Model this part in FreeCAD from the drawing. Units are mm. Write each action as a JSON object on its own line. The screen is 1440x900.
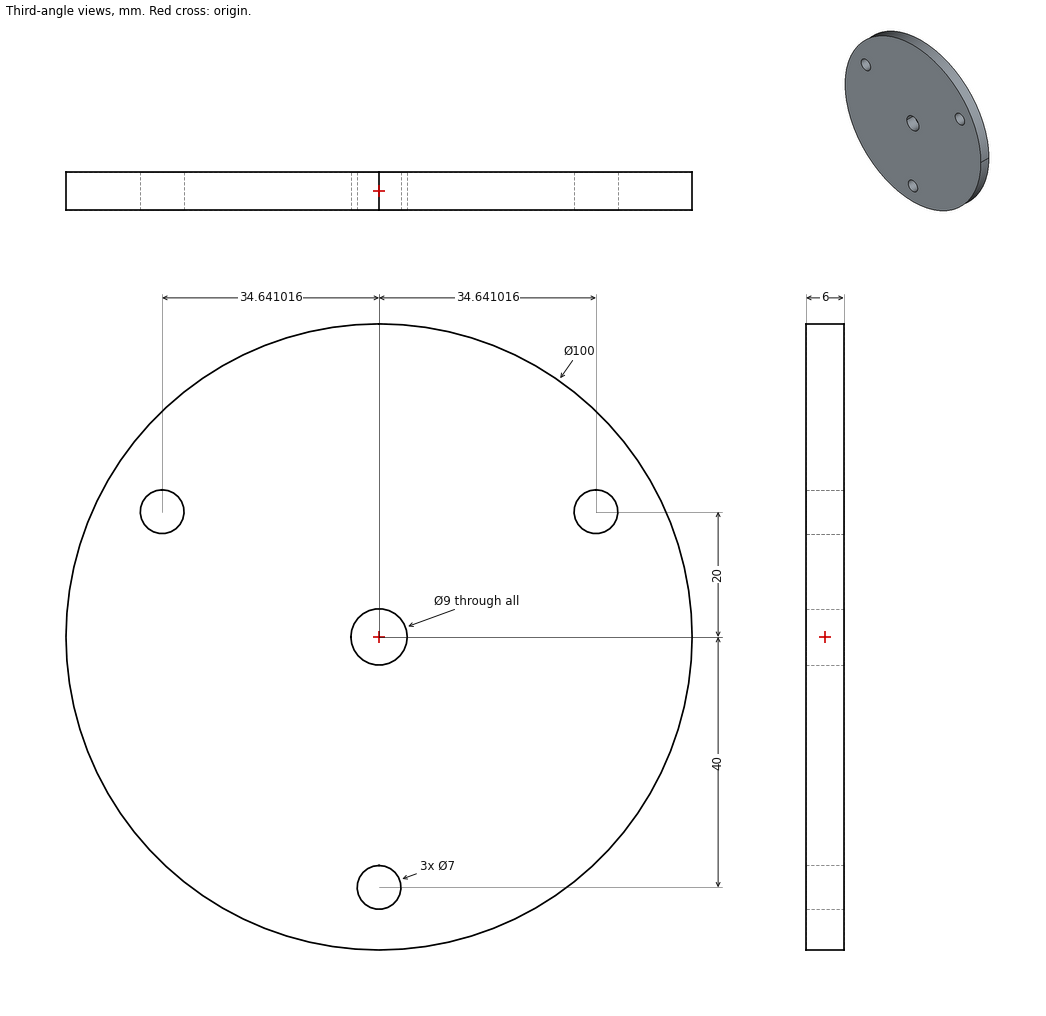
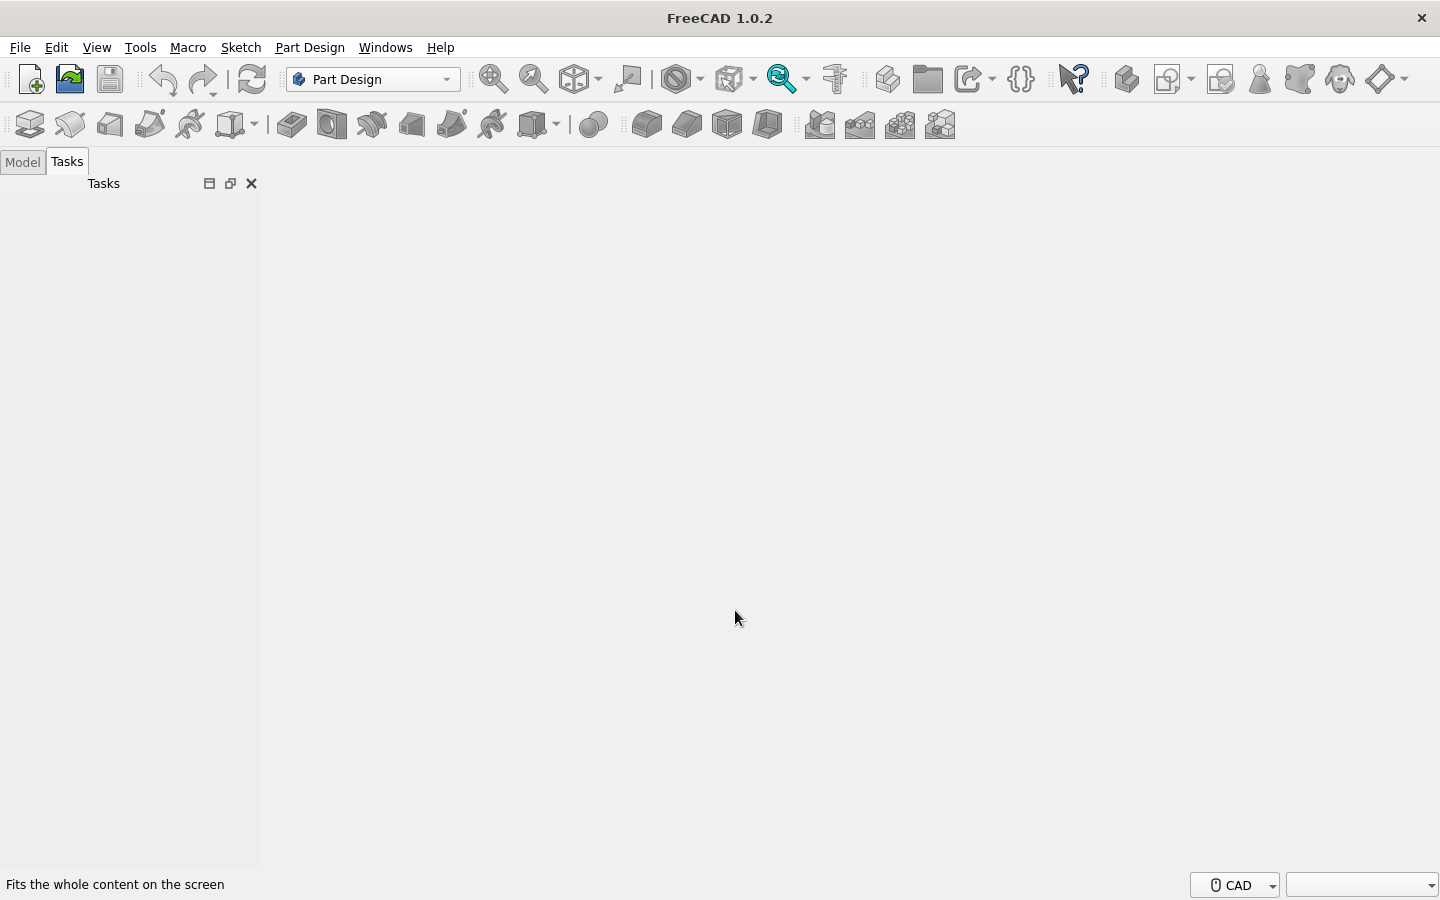
{"action": "left_click", "coordinate": [30, 80]}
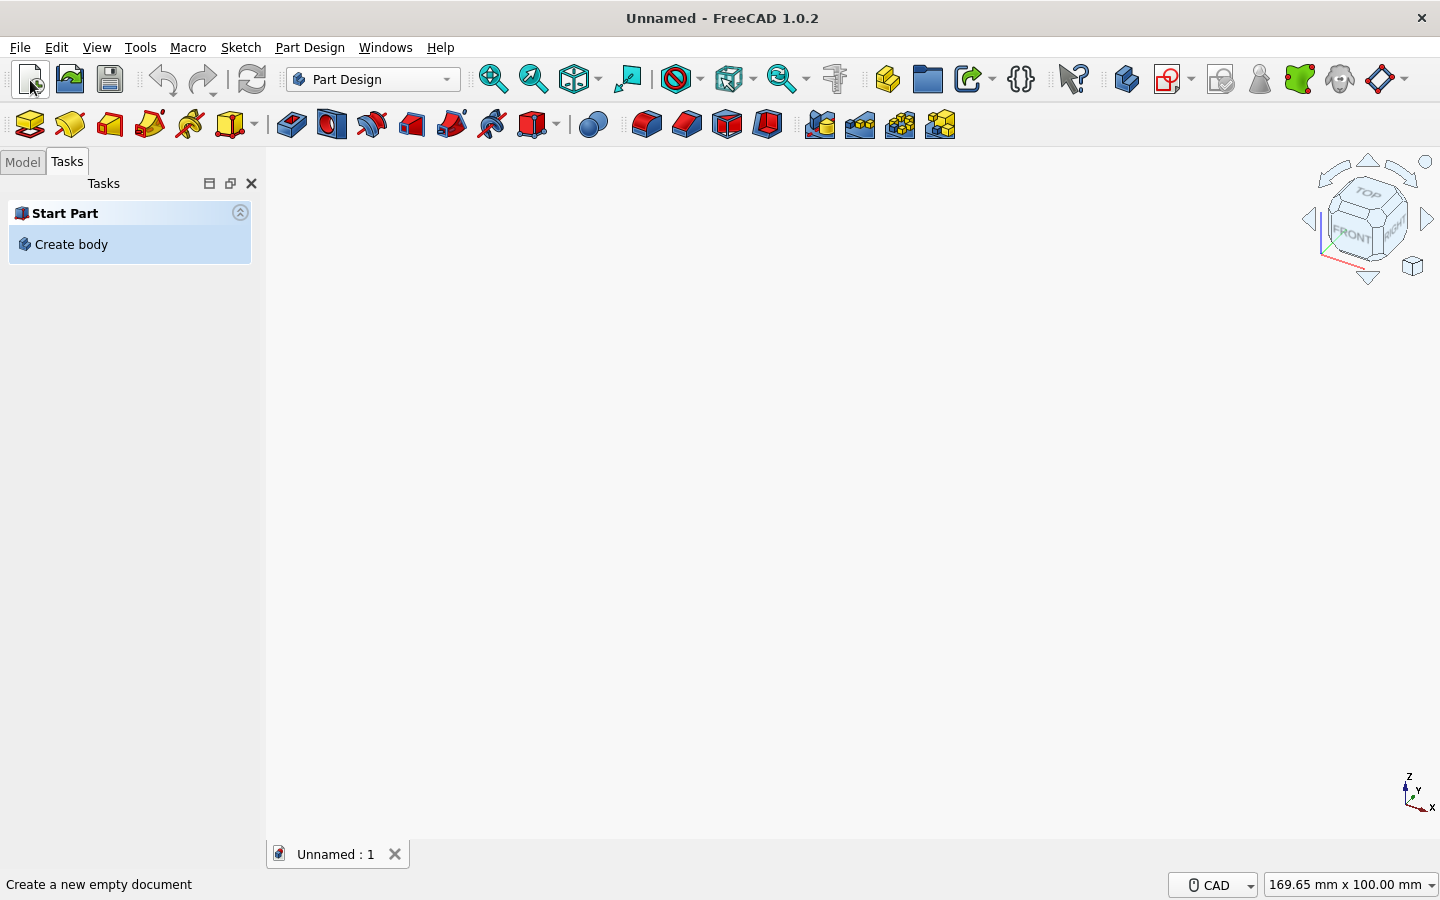
{"action": "left_click", "coordinate": [1168, 80]}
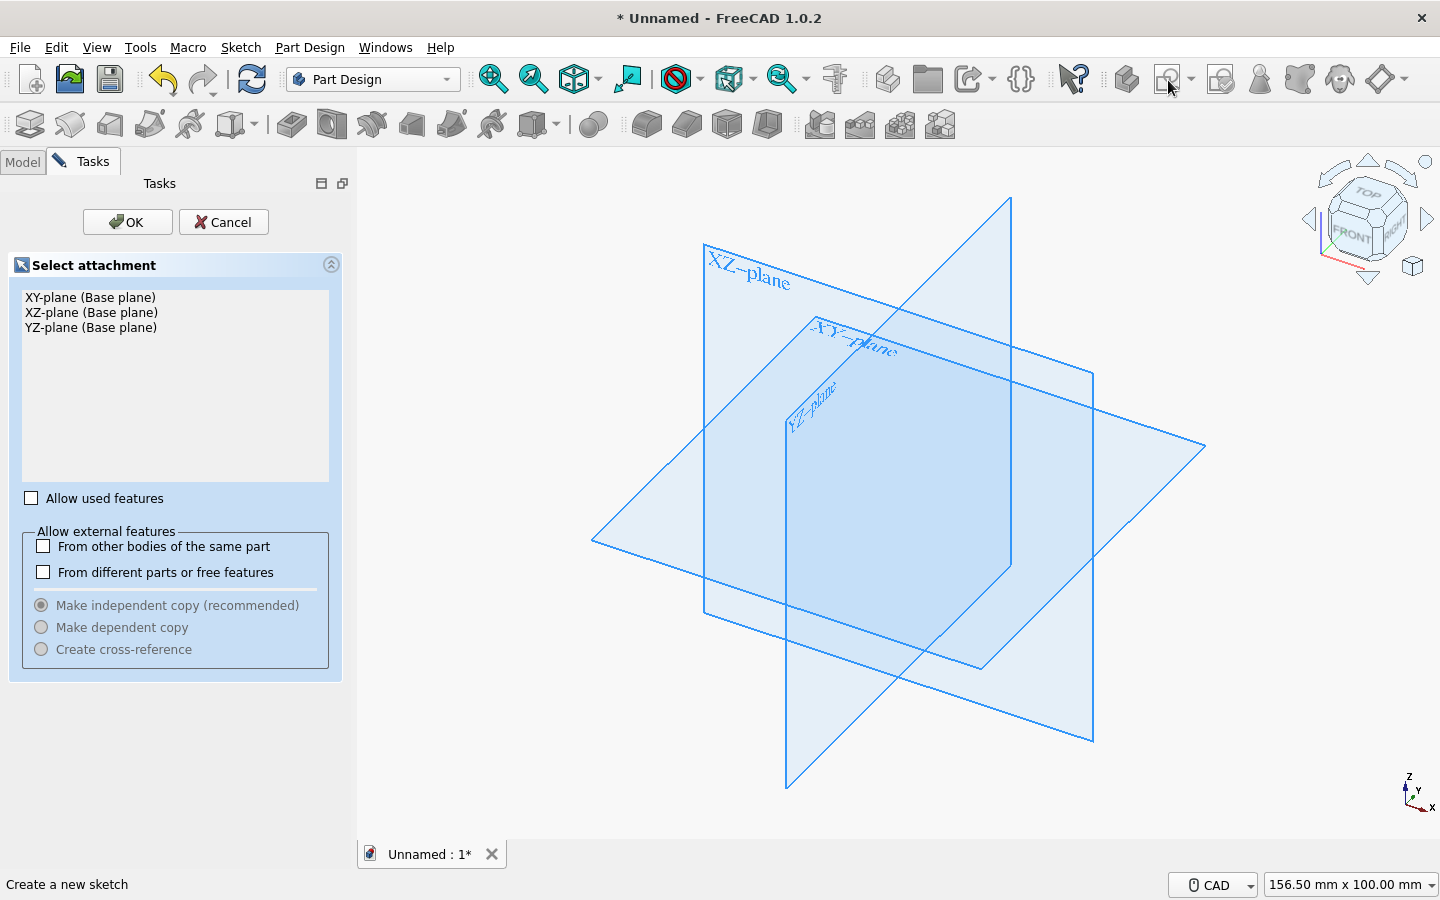
{"action": "left_click", "coordinate": [82, 312]}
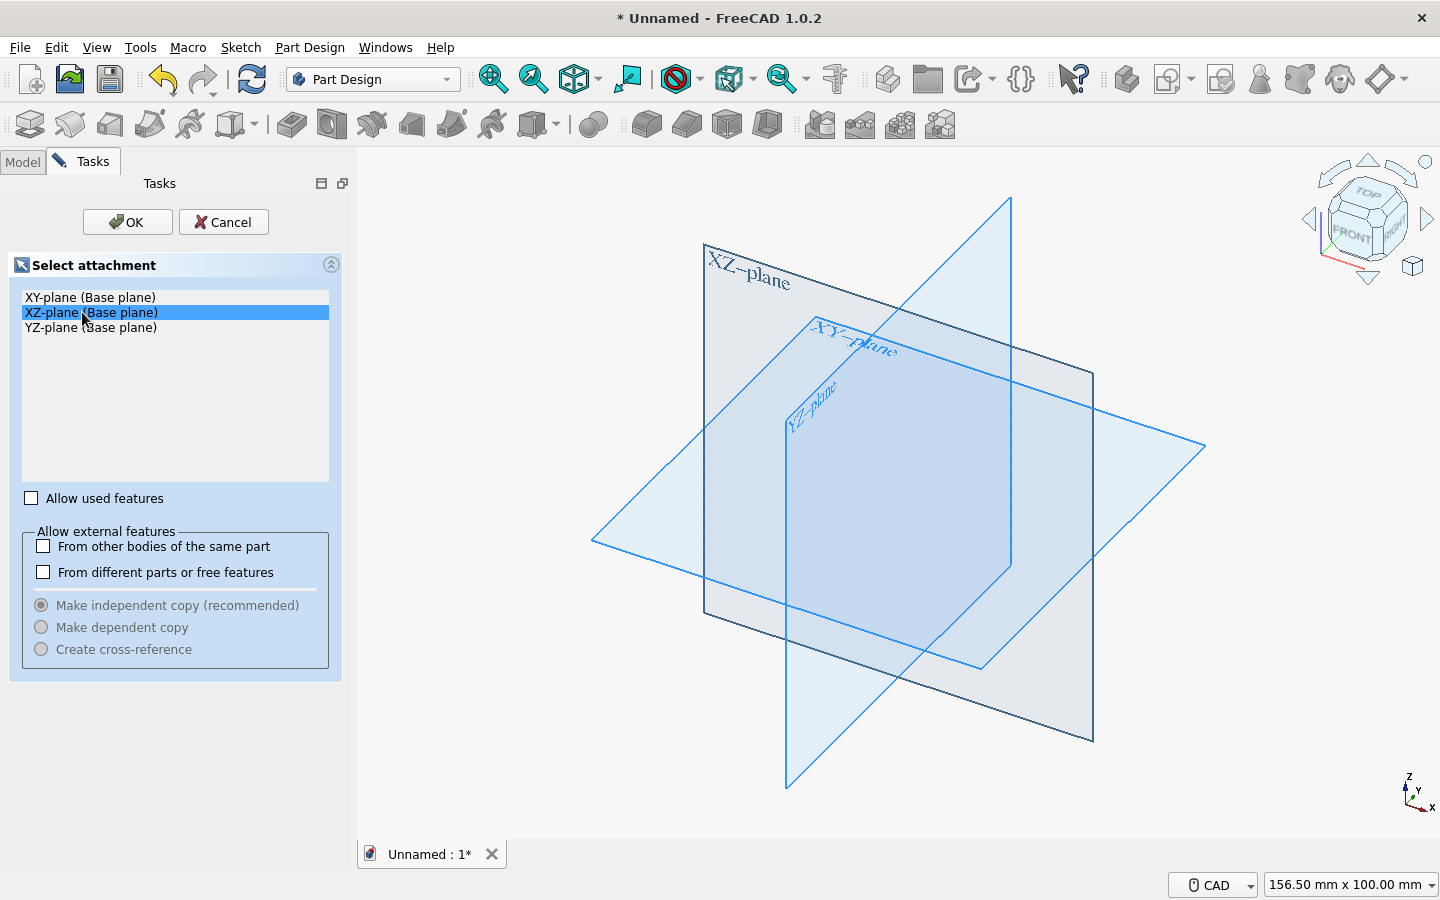
{"action": "left_click", "coordinate": [128, 222]}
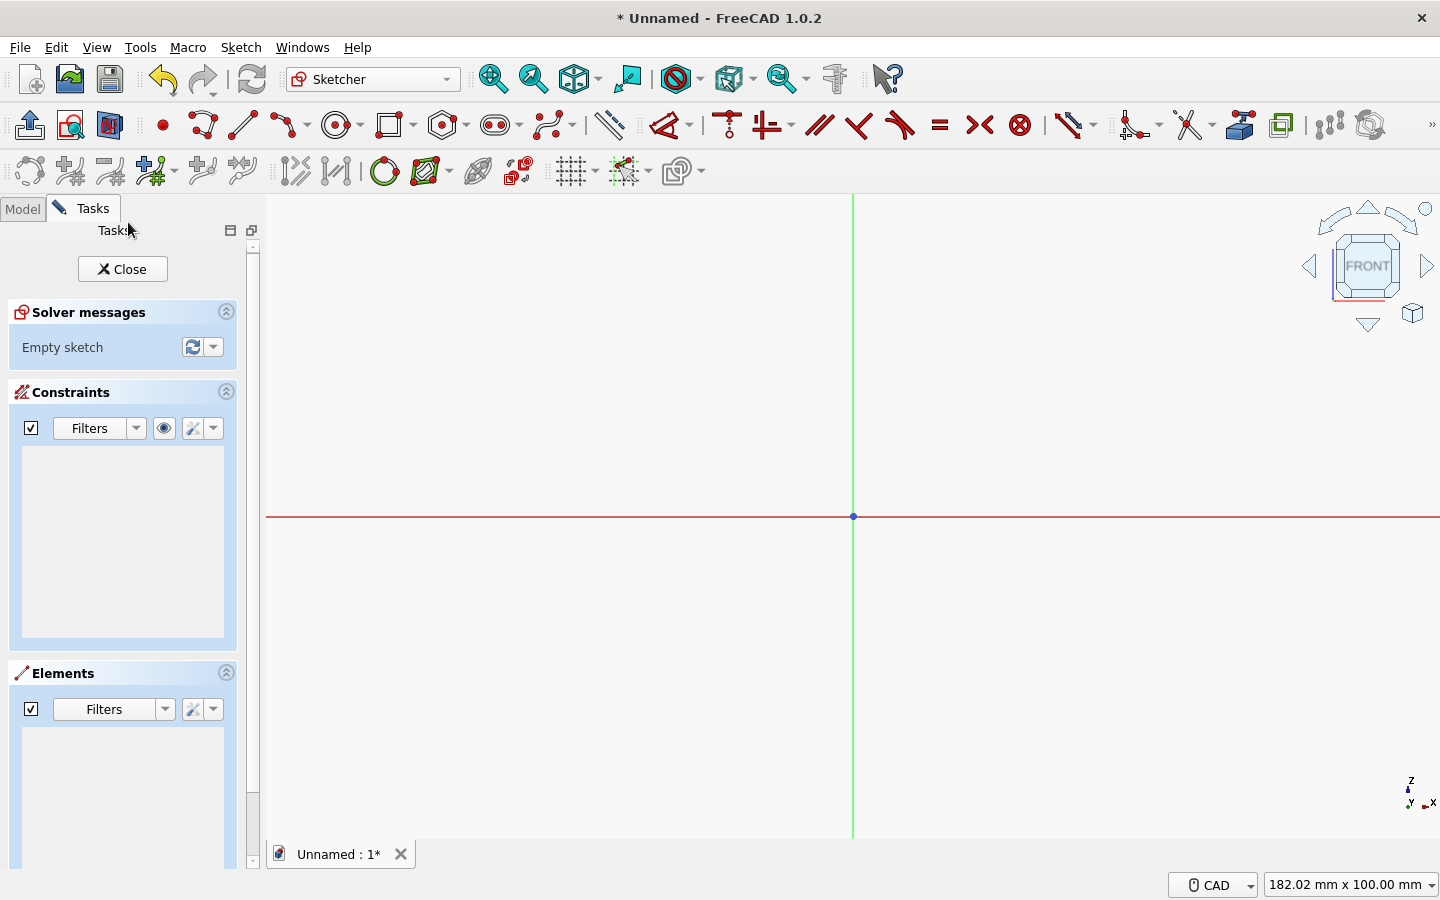
{"action": "scroll", "coordinate": [645, 516], "scroll_direction": "down", "scroll_amount": 2}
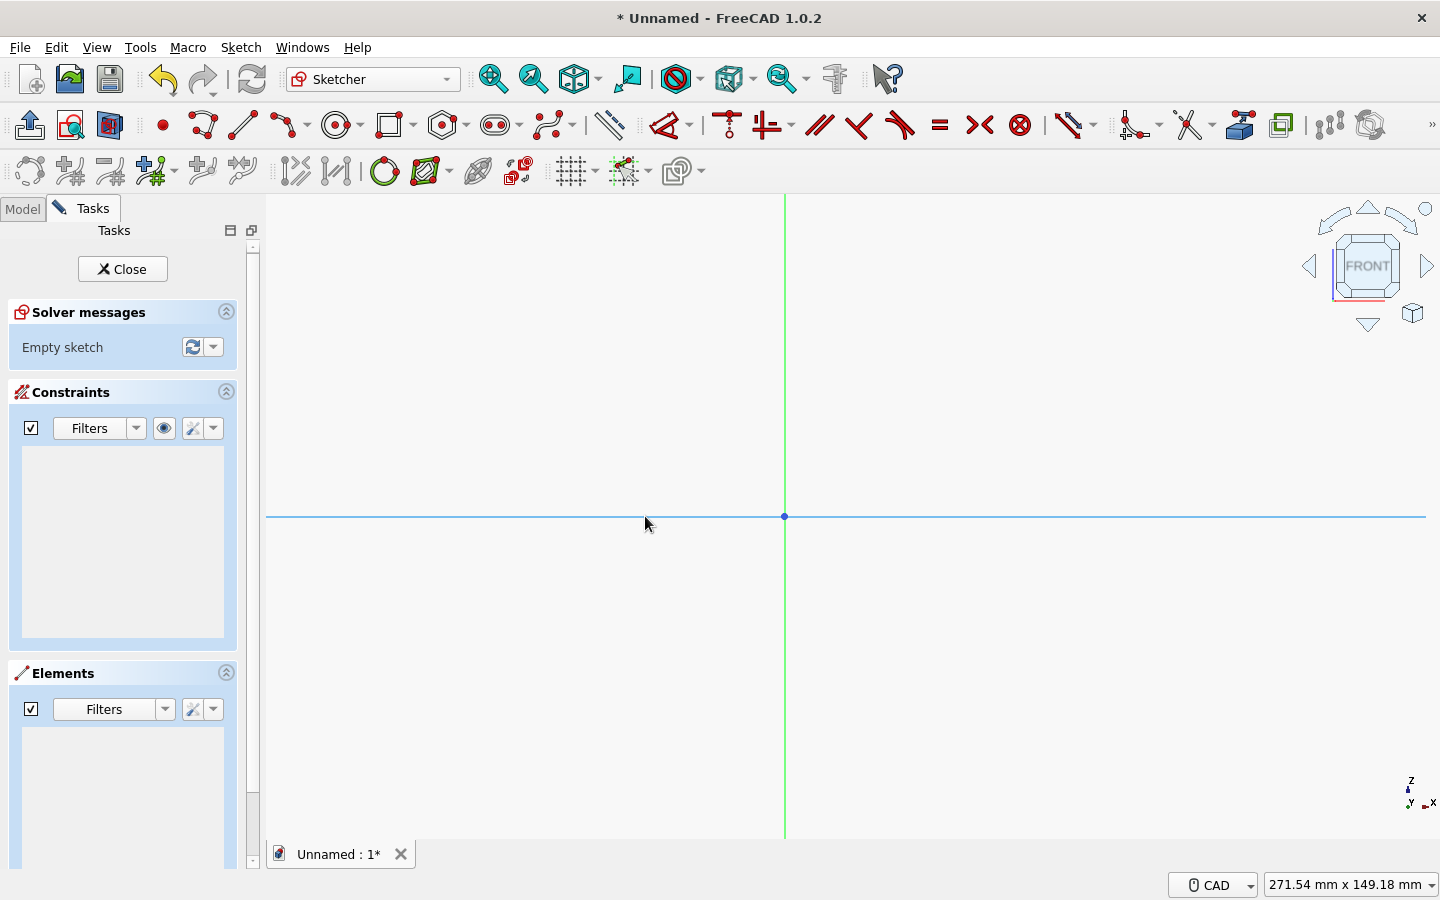
{"action": "left_click", "coordinate": [336, 126]}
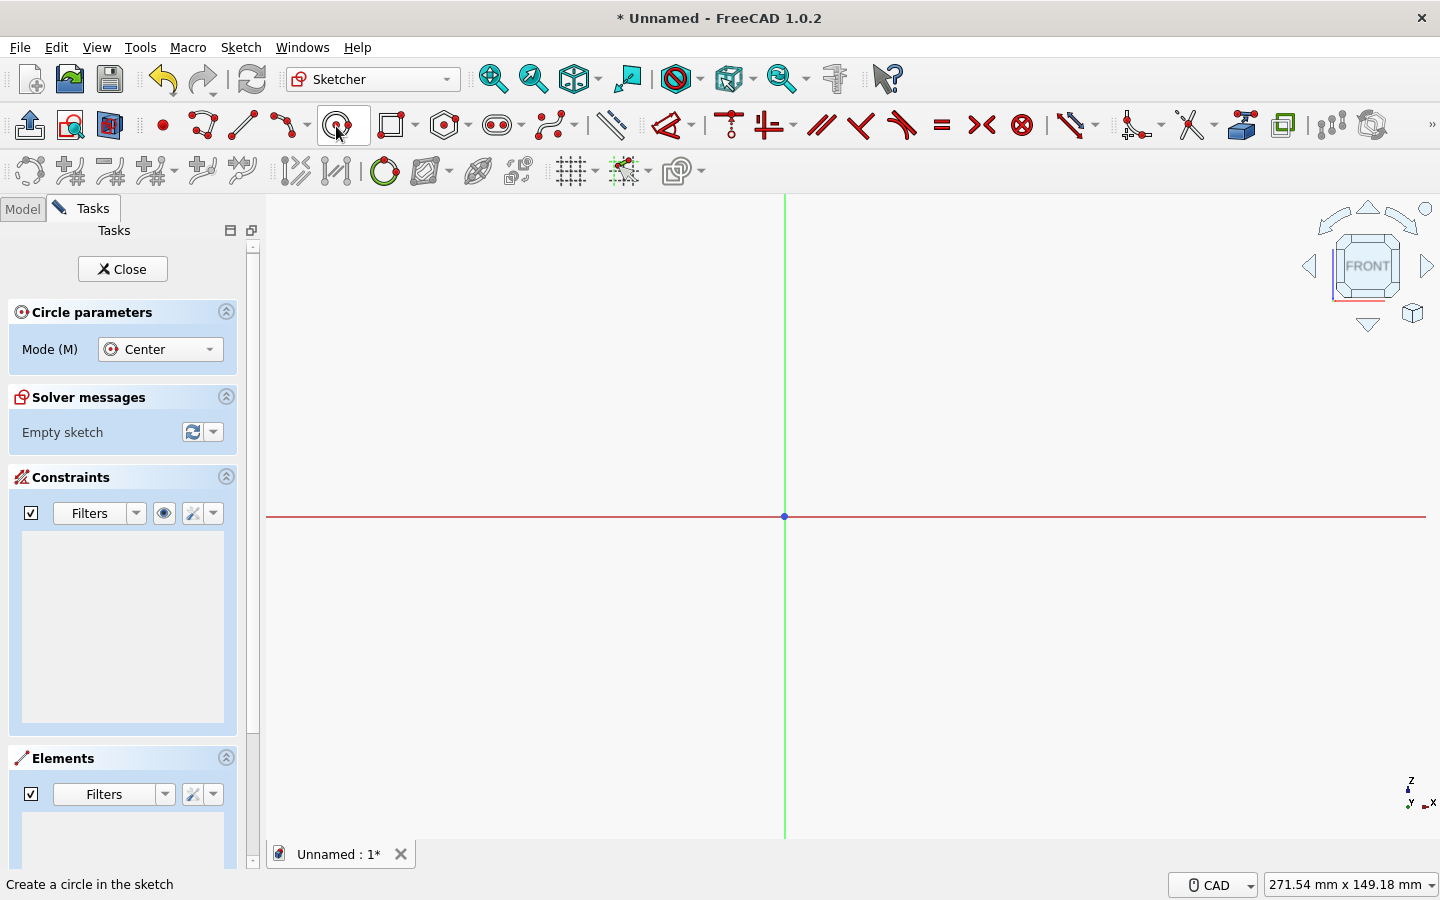
{"action": "left_click", "coordinate": [785, 516]}
{"action": "mouse_move", "coordinate": [937, 364]}